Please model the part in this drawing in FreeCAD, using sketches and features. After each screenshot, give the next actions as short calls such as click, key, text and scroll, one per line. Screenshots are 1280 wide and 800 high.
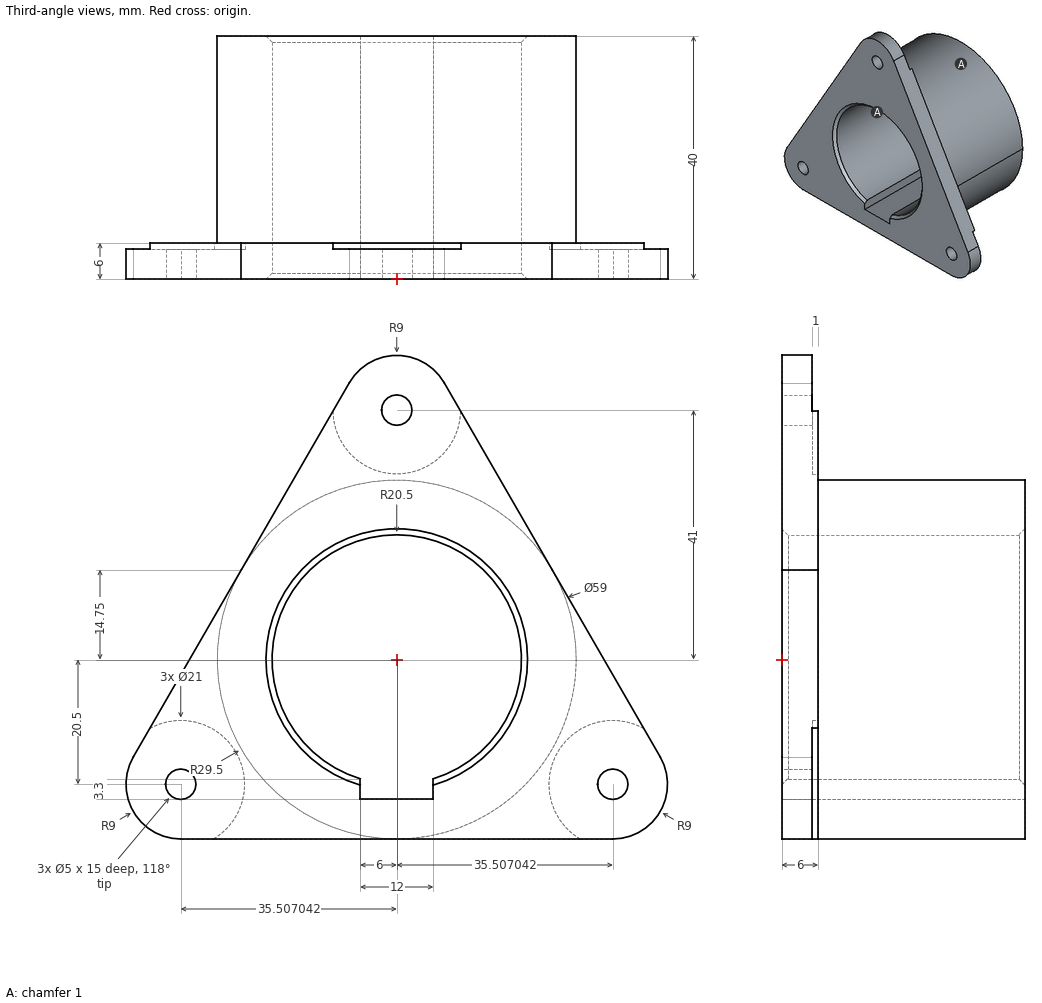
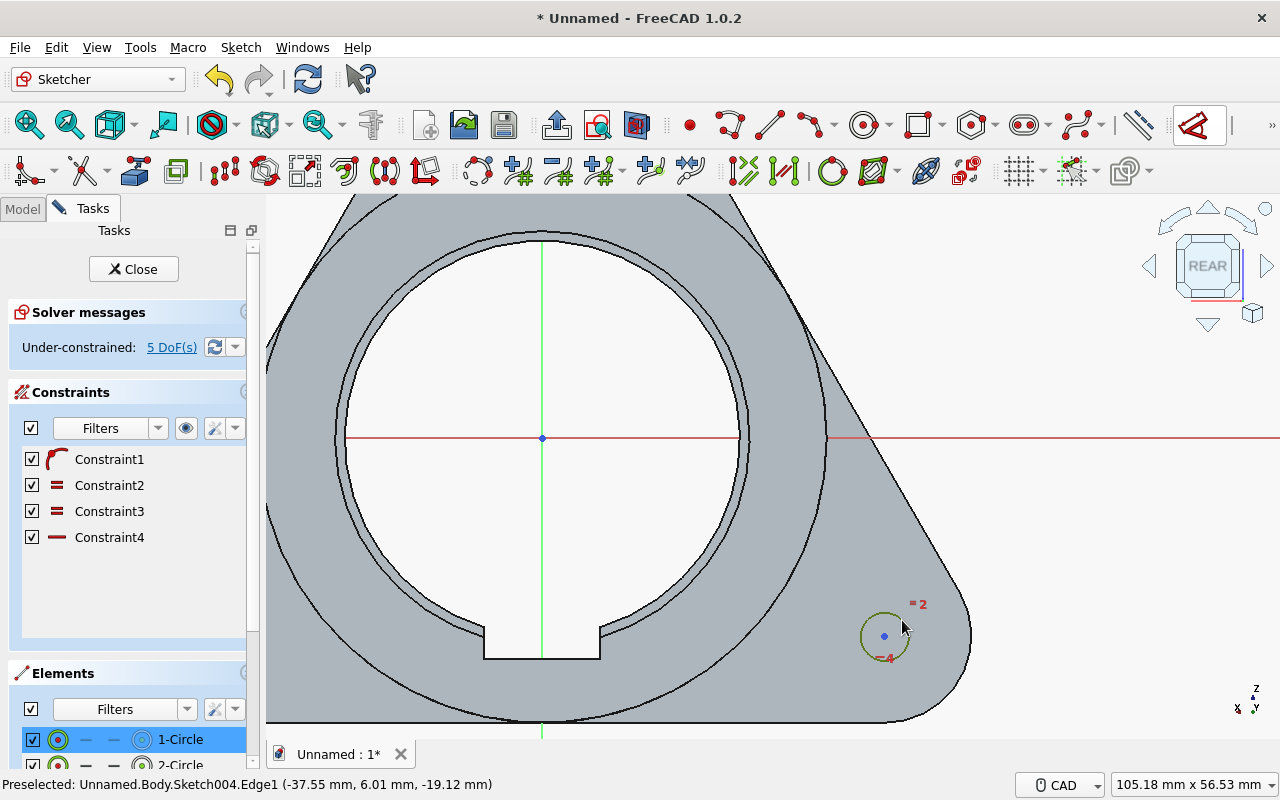
key(k)
key(o)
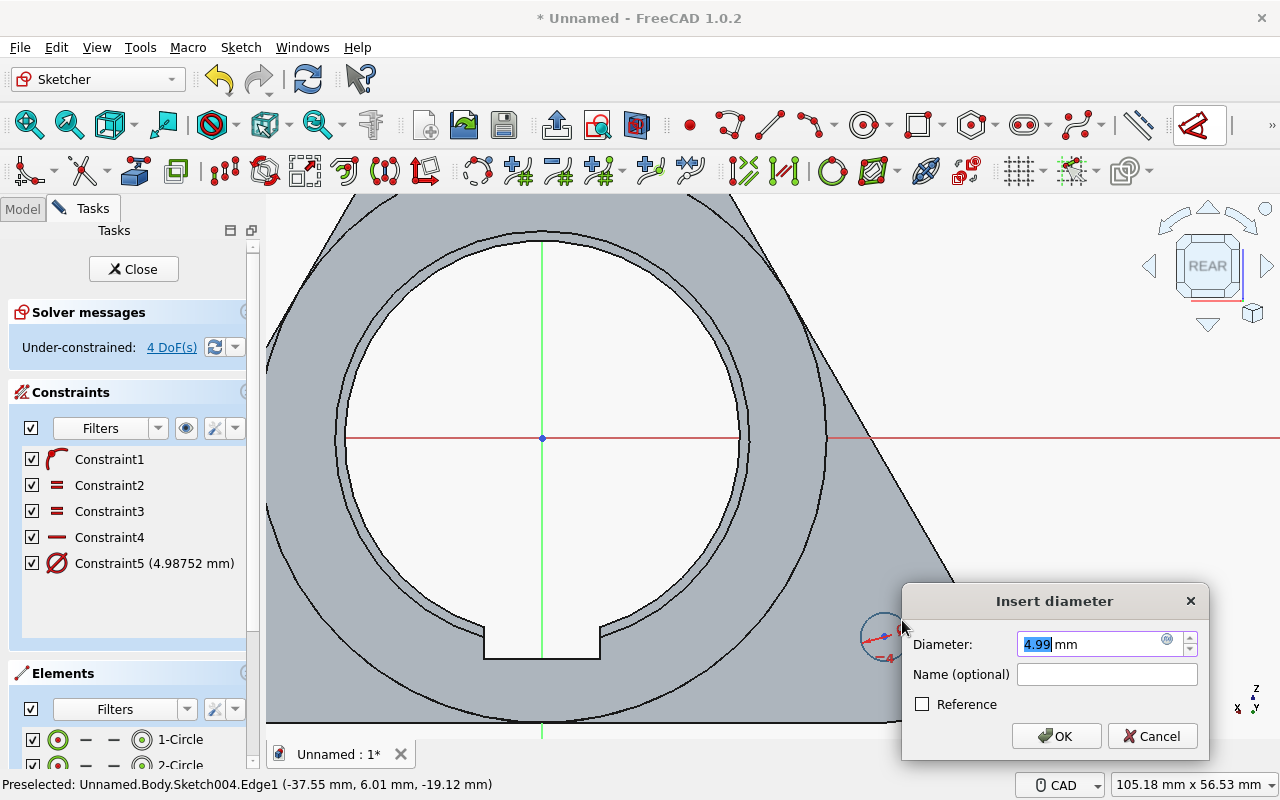
text(5)
key(Return)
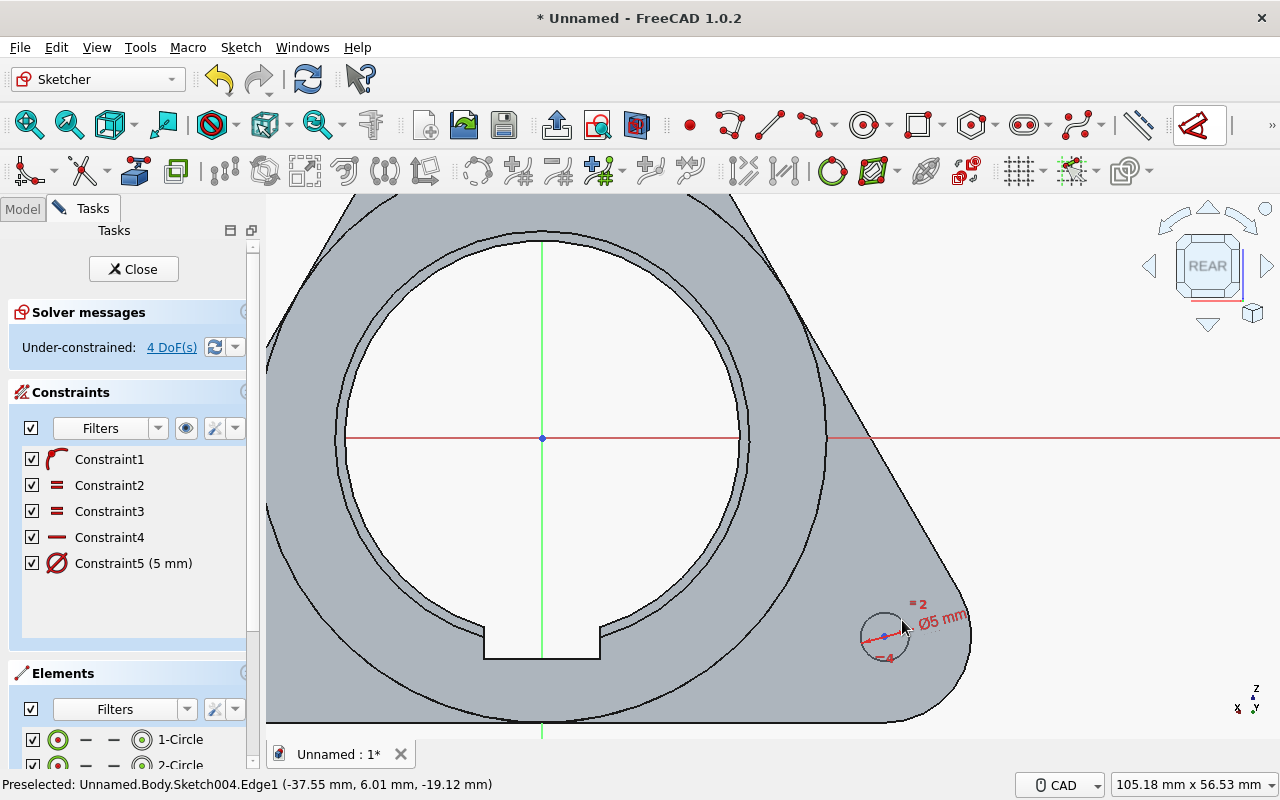
scroll(902, 621, down, 3)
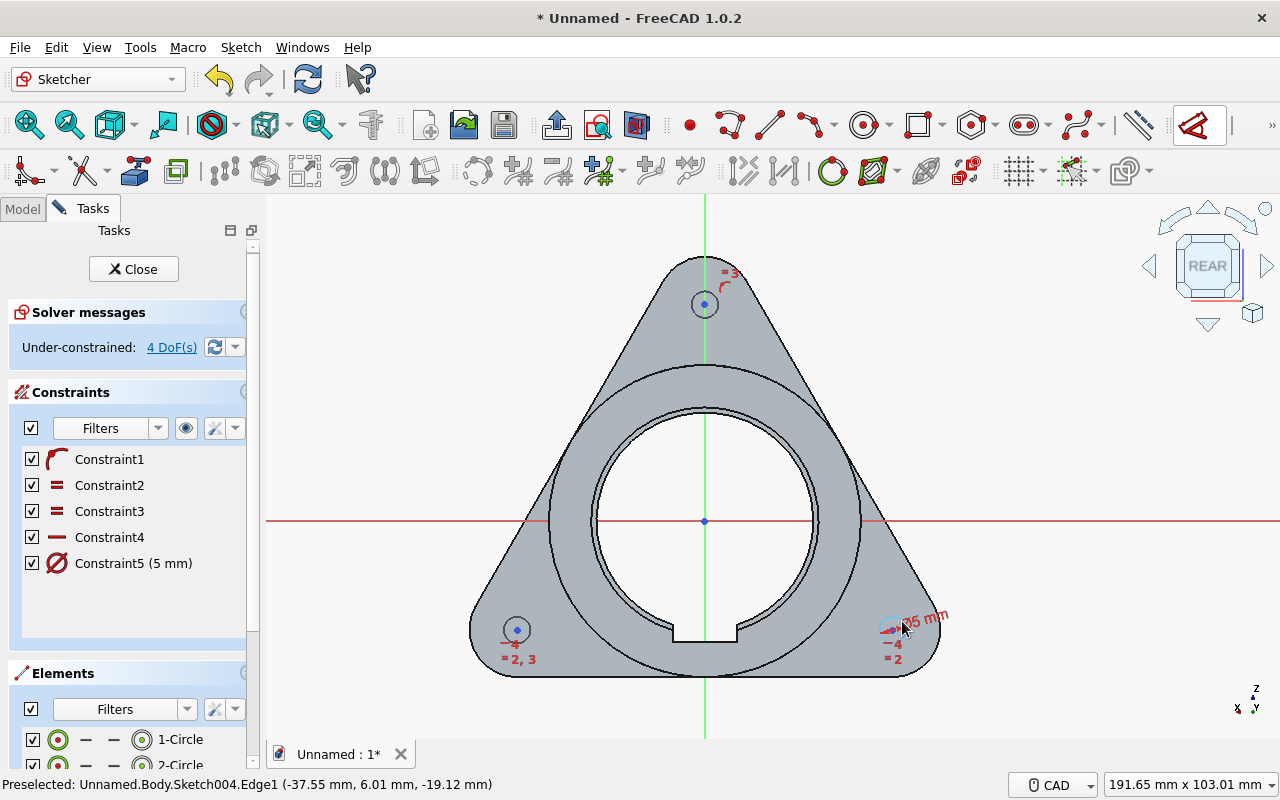
click(705, 305)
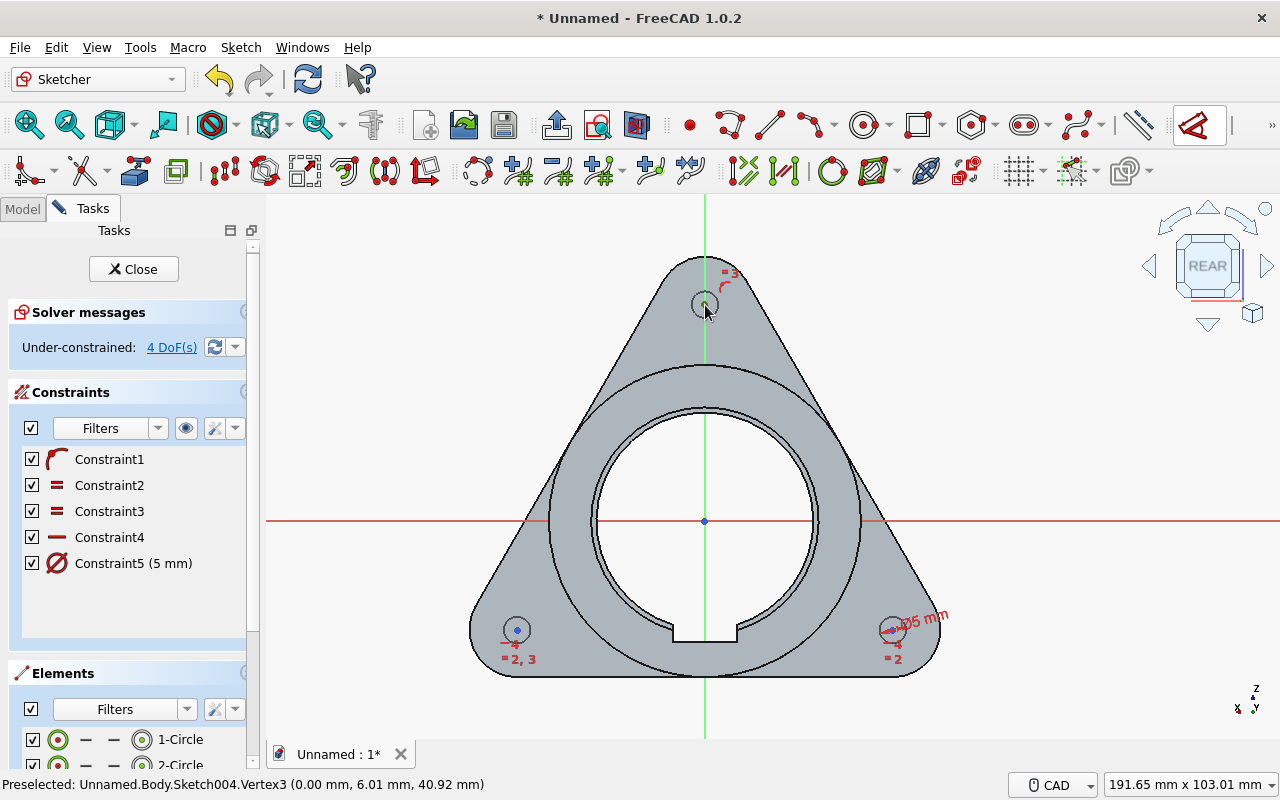
click(1220, 126)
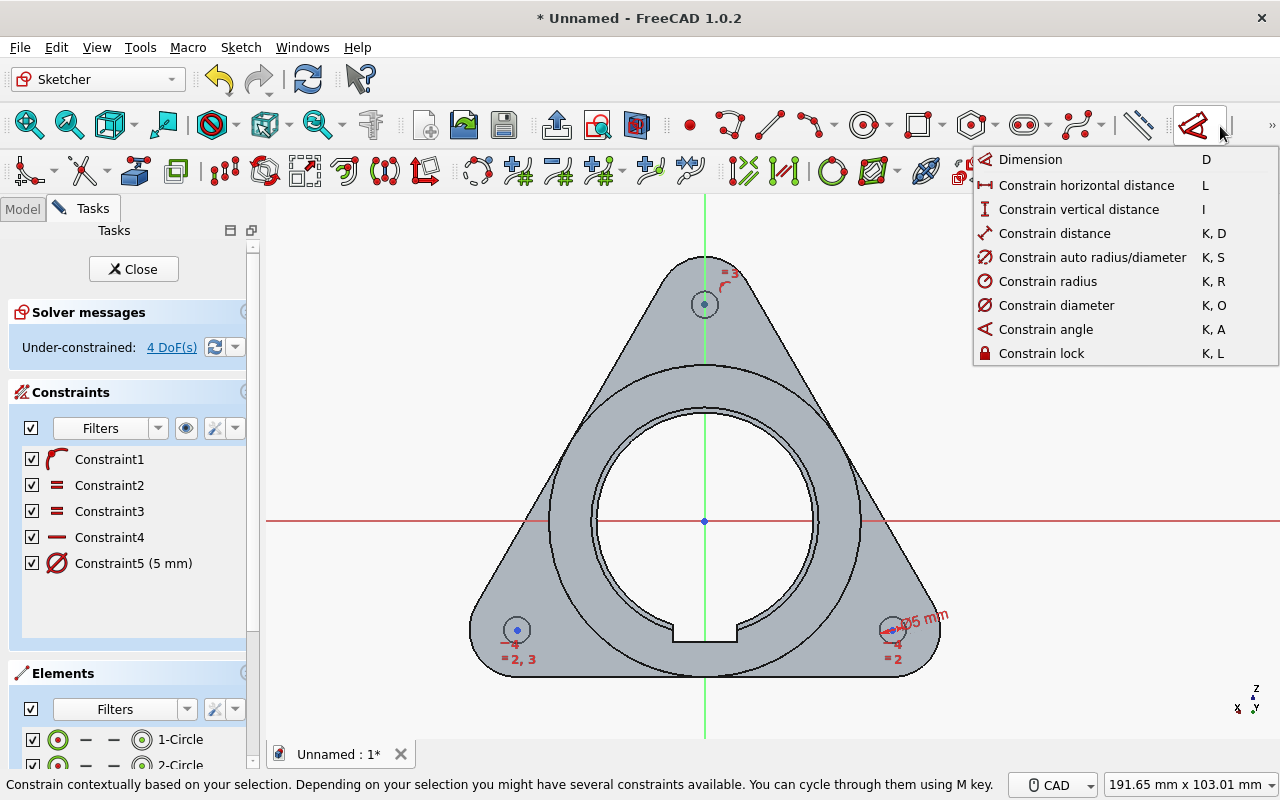
click(1126, 209)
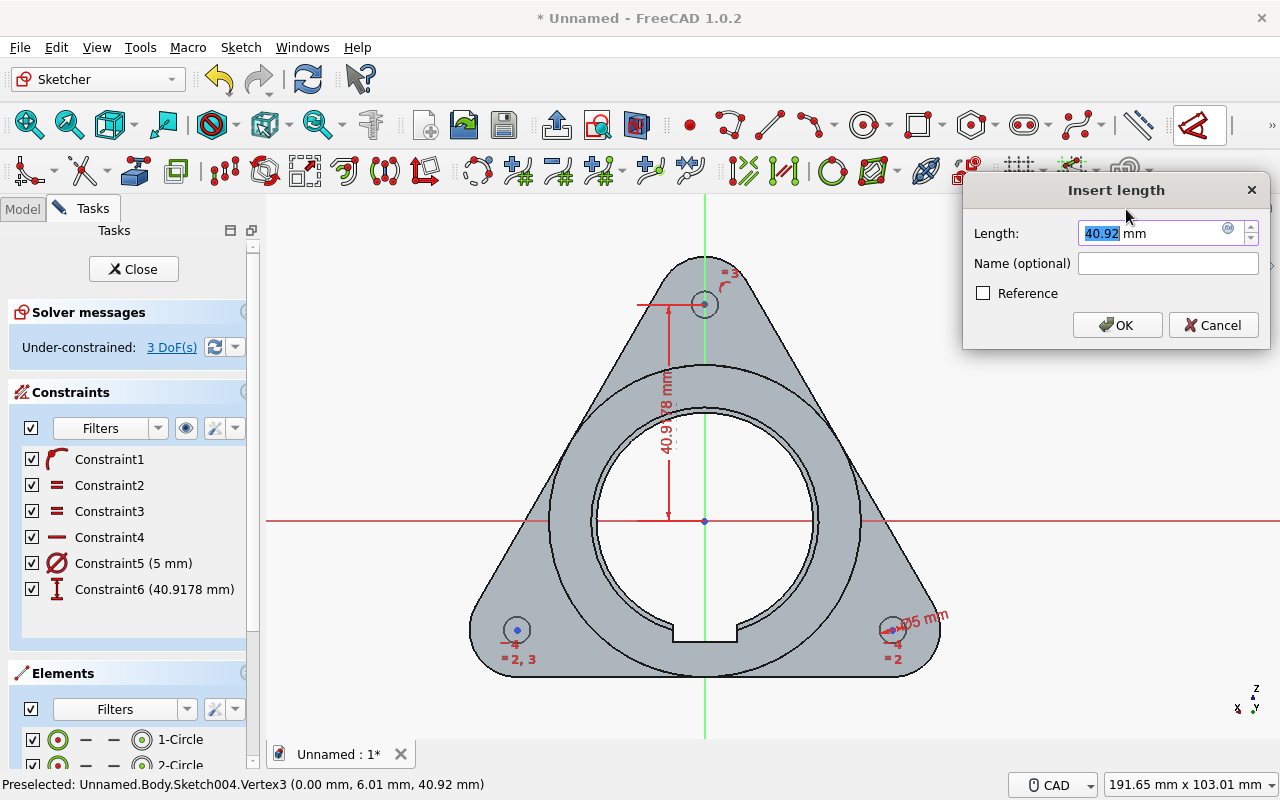
text(41)
key(Return)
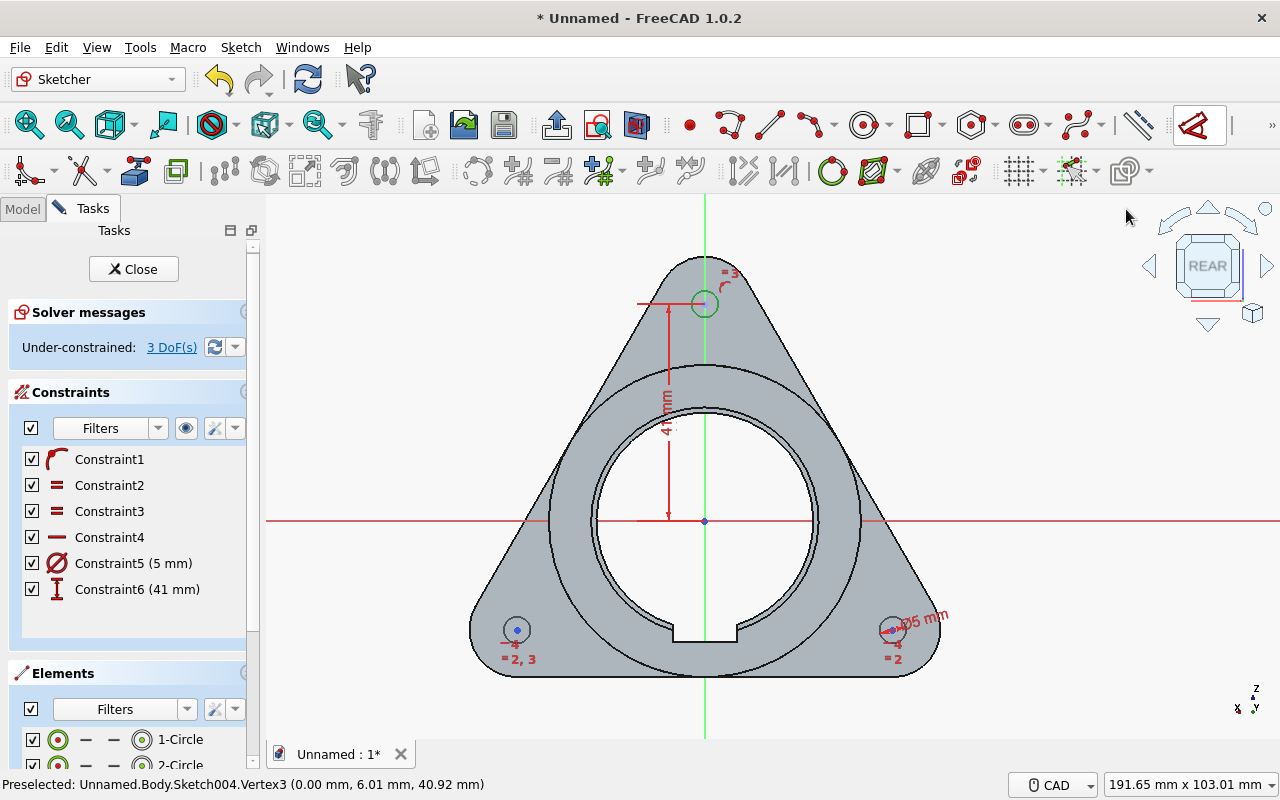
click(893, 630)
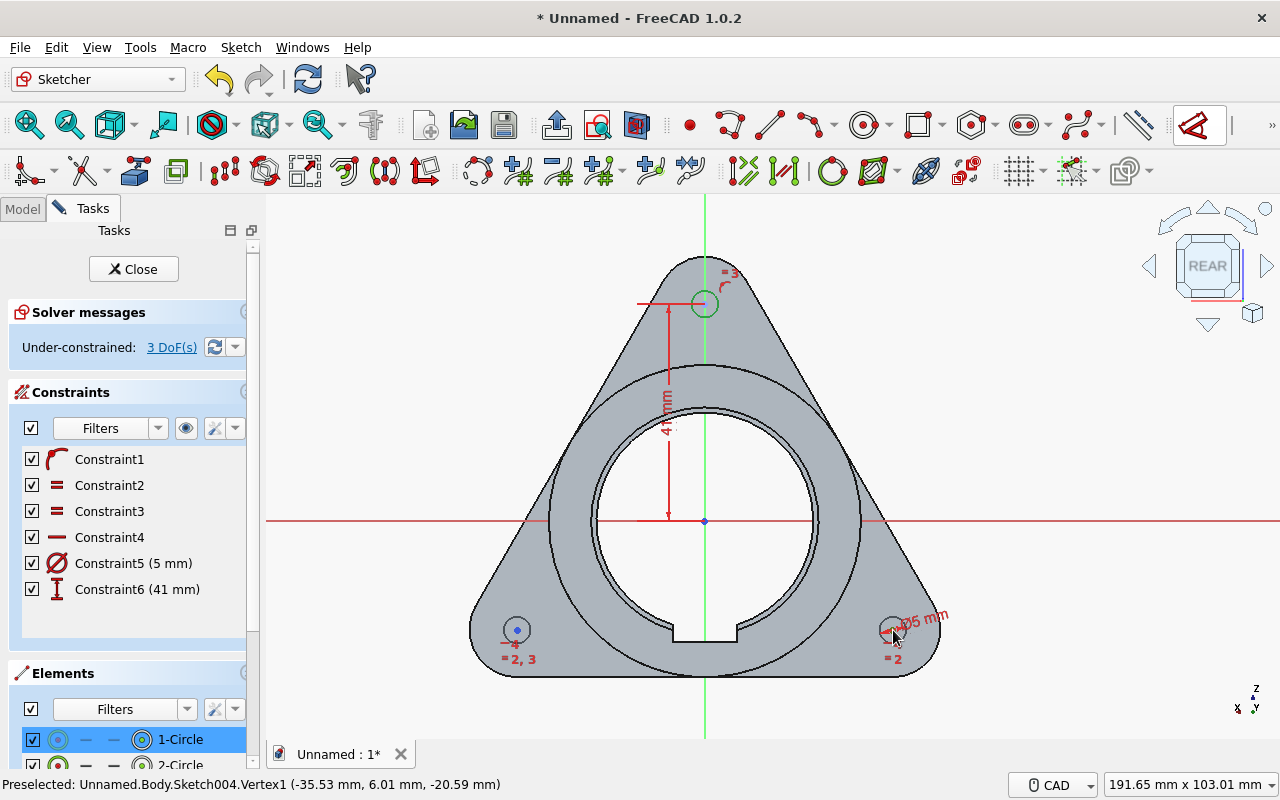
click(1220, 126)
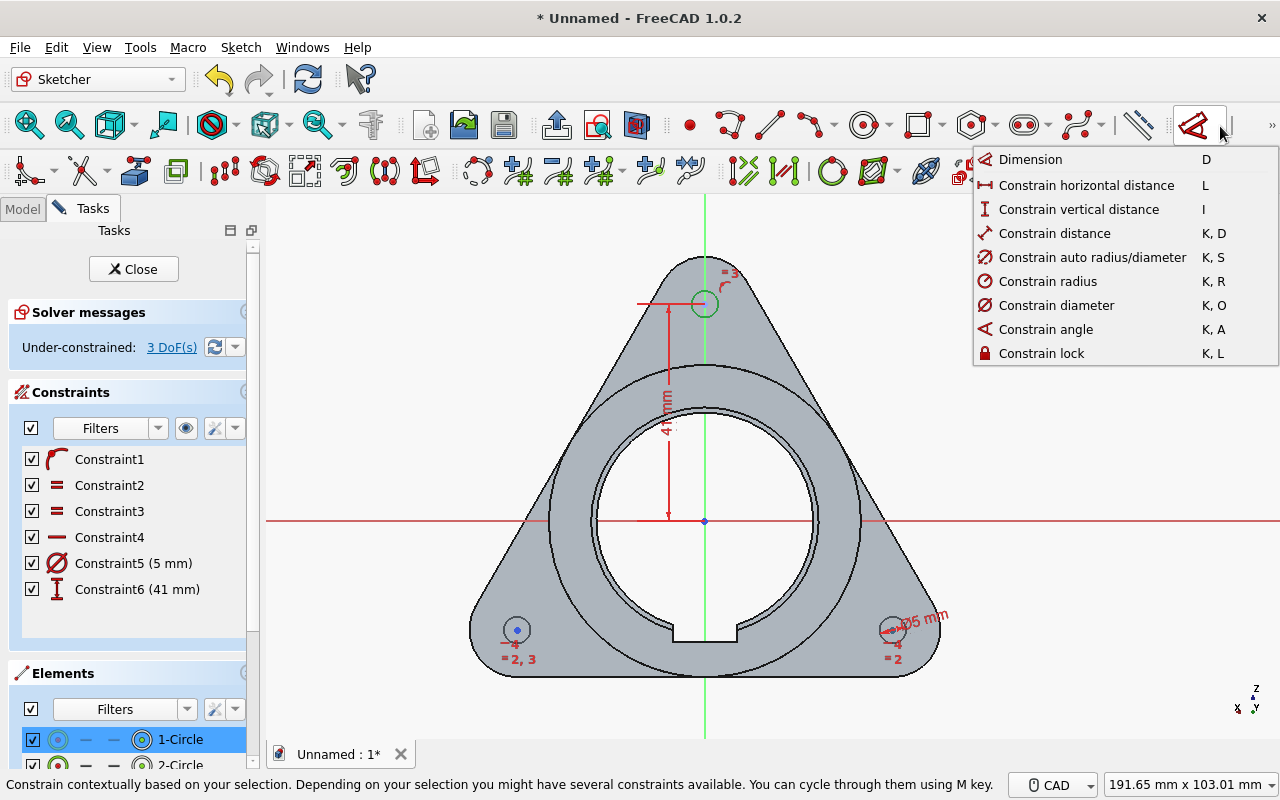
click(1126, 209)